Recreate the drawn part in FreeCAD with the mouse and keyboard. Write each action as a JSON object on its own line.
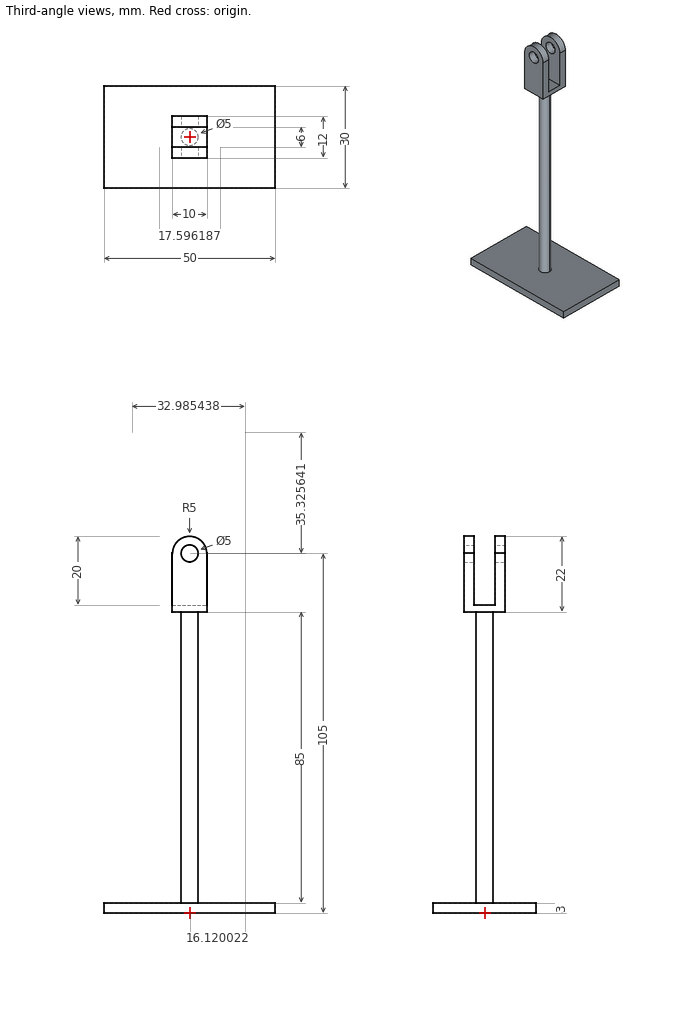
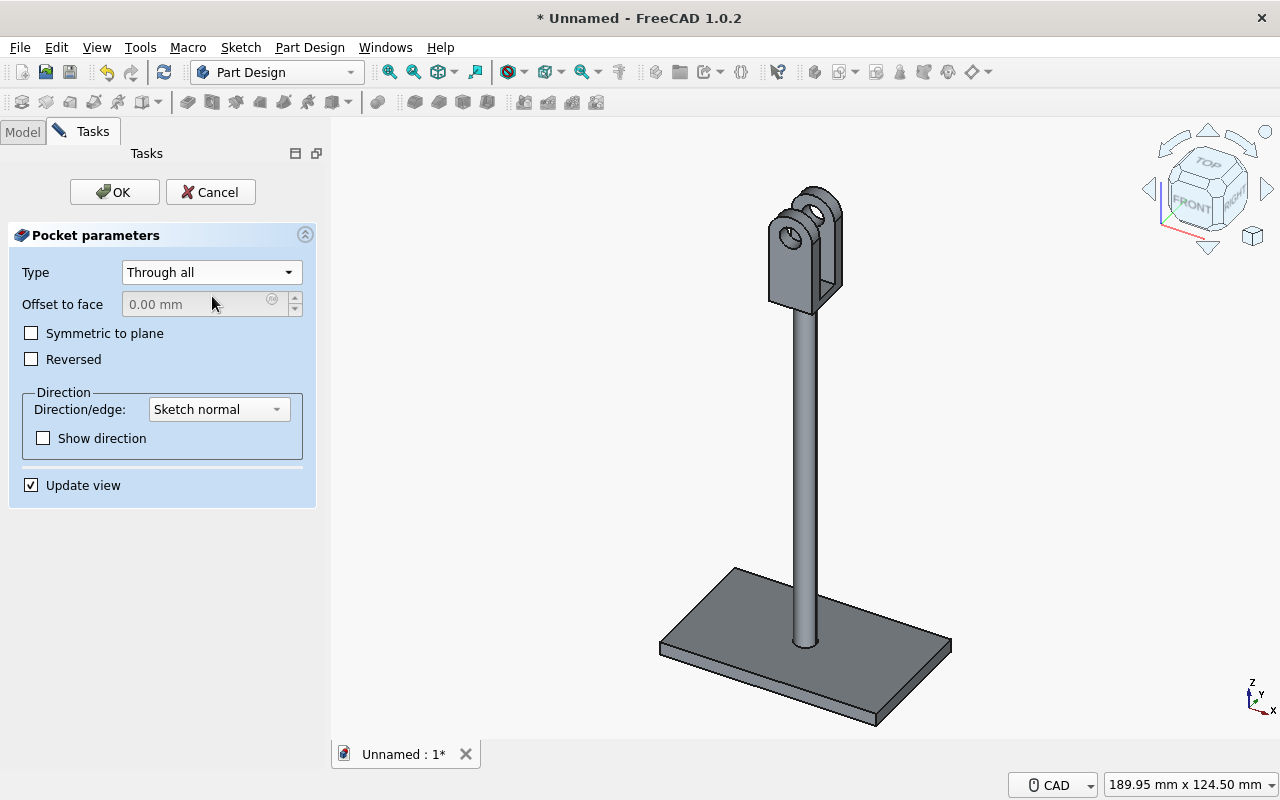
{"action": "left_click", "coordinate": [115, 192]}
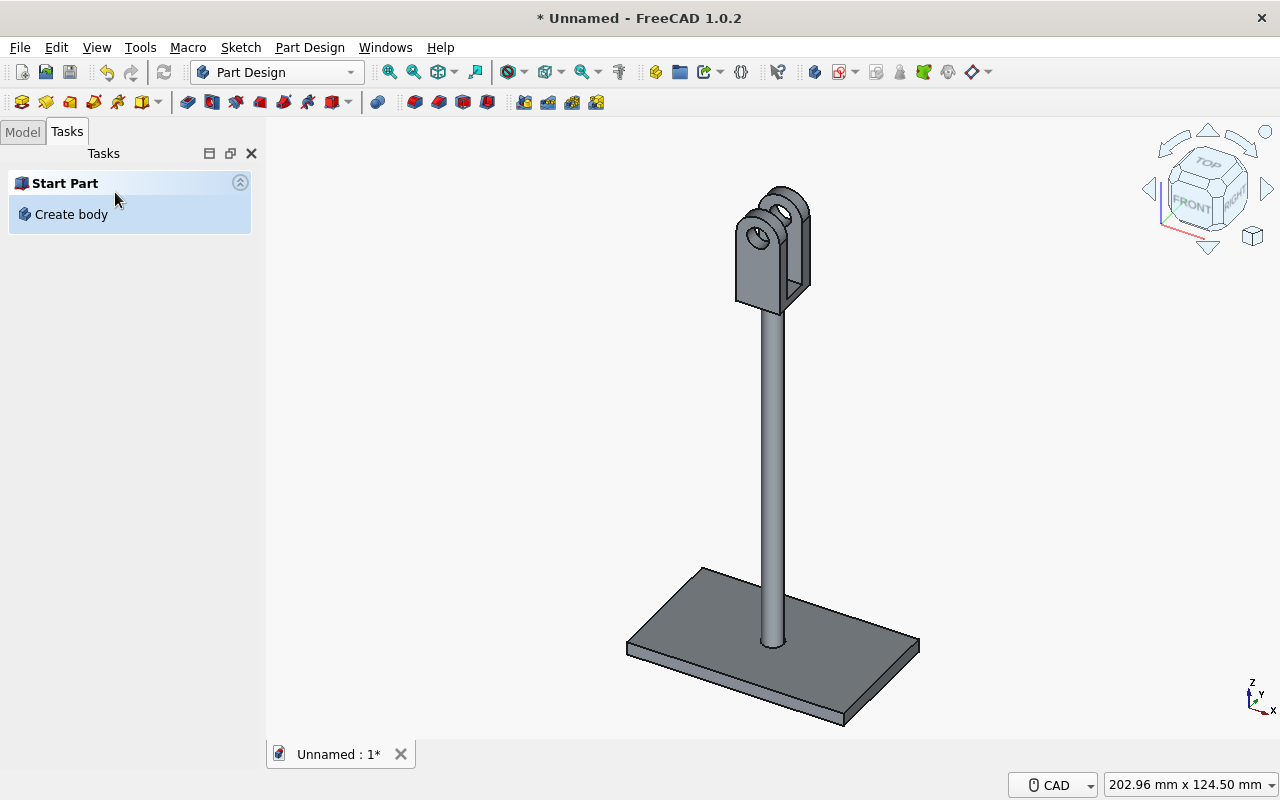
{"action": "key", "text": "0"}